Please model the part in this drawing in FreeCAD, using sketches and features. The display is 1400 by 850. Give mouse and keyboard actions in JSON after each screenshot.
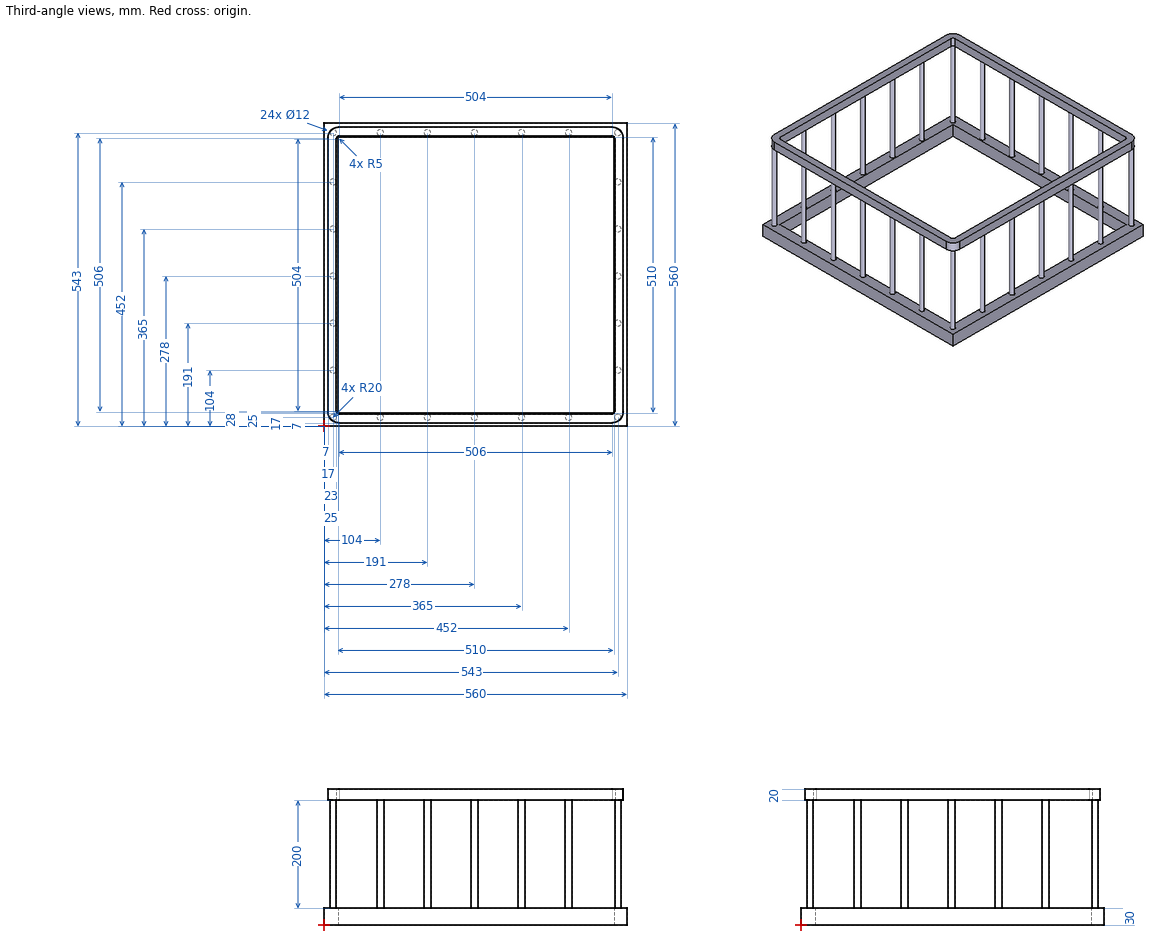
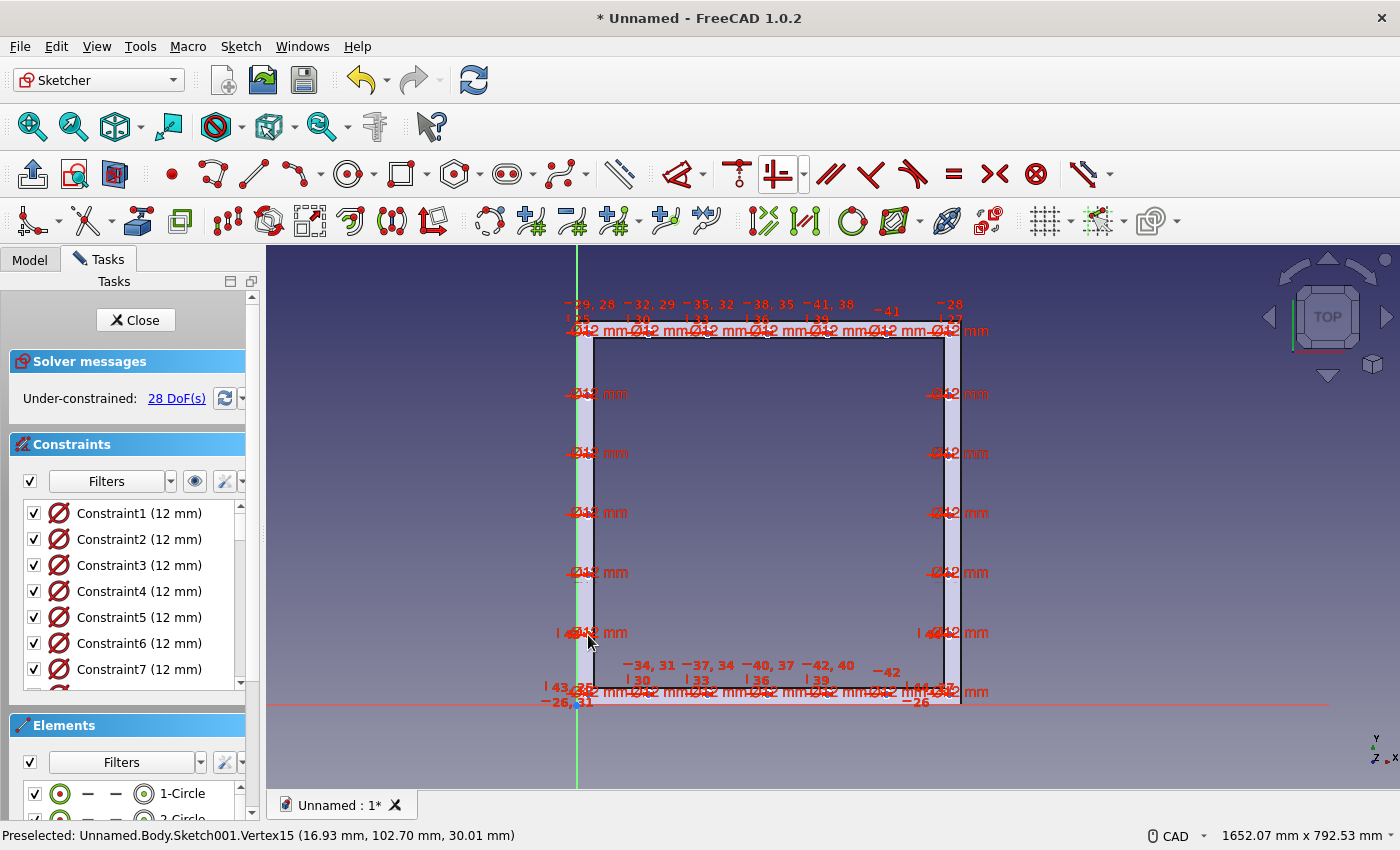
{"action": "left_click", "coordinate": [588, 575]}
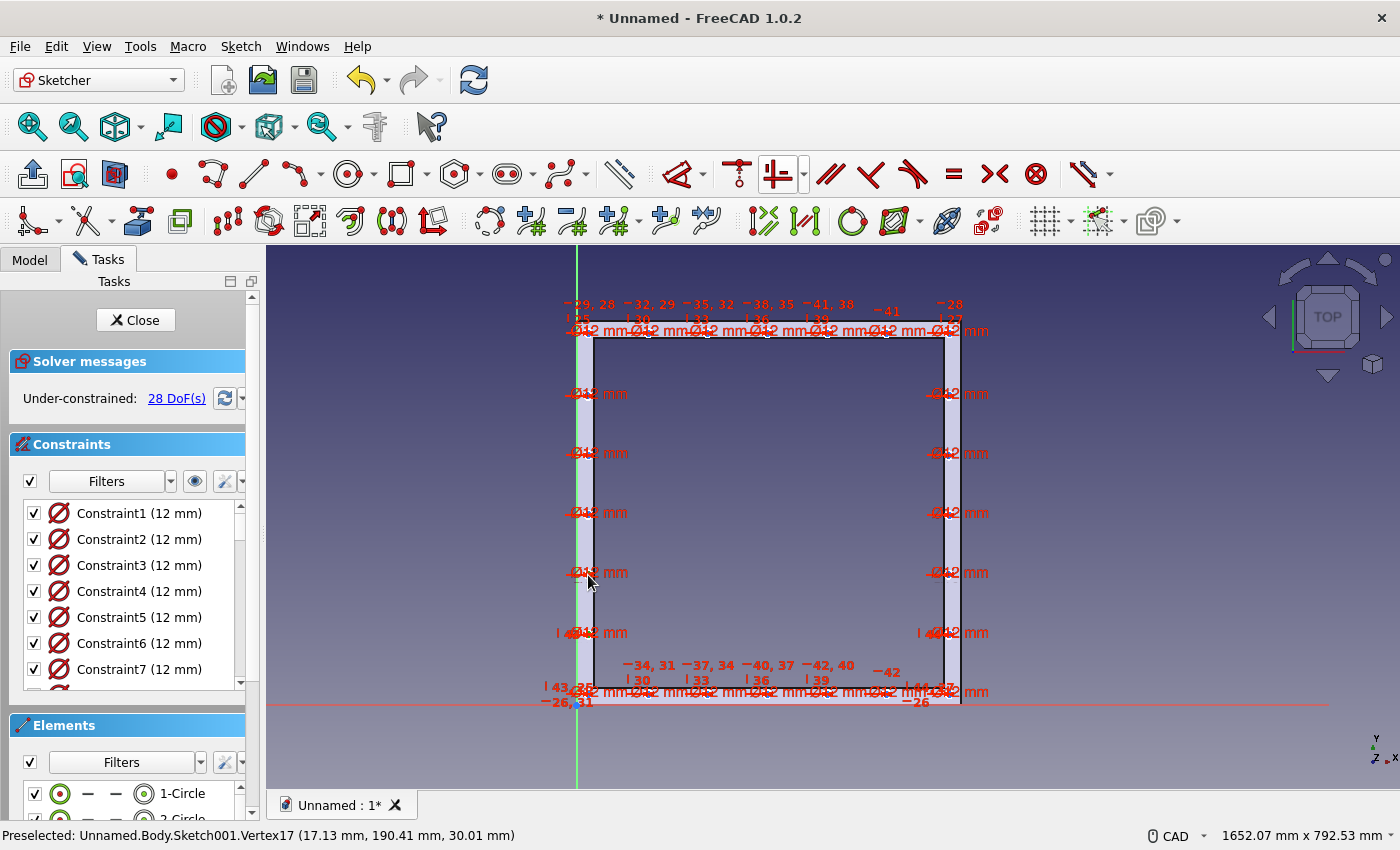
{"action": "left_click", "coordinate": [804, 174]}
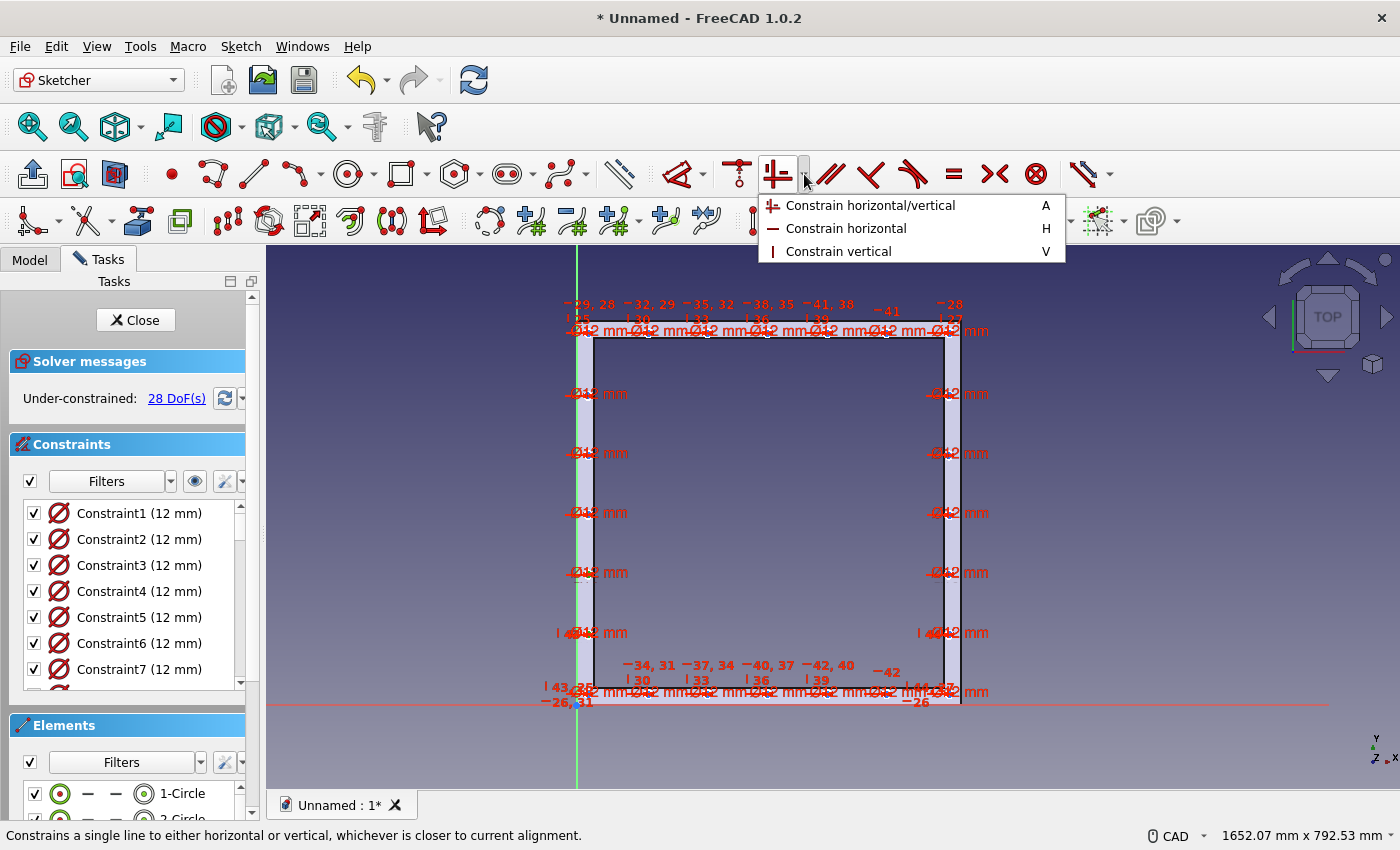
{"action": "left_click", "coordinate": [912, 252]}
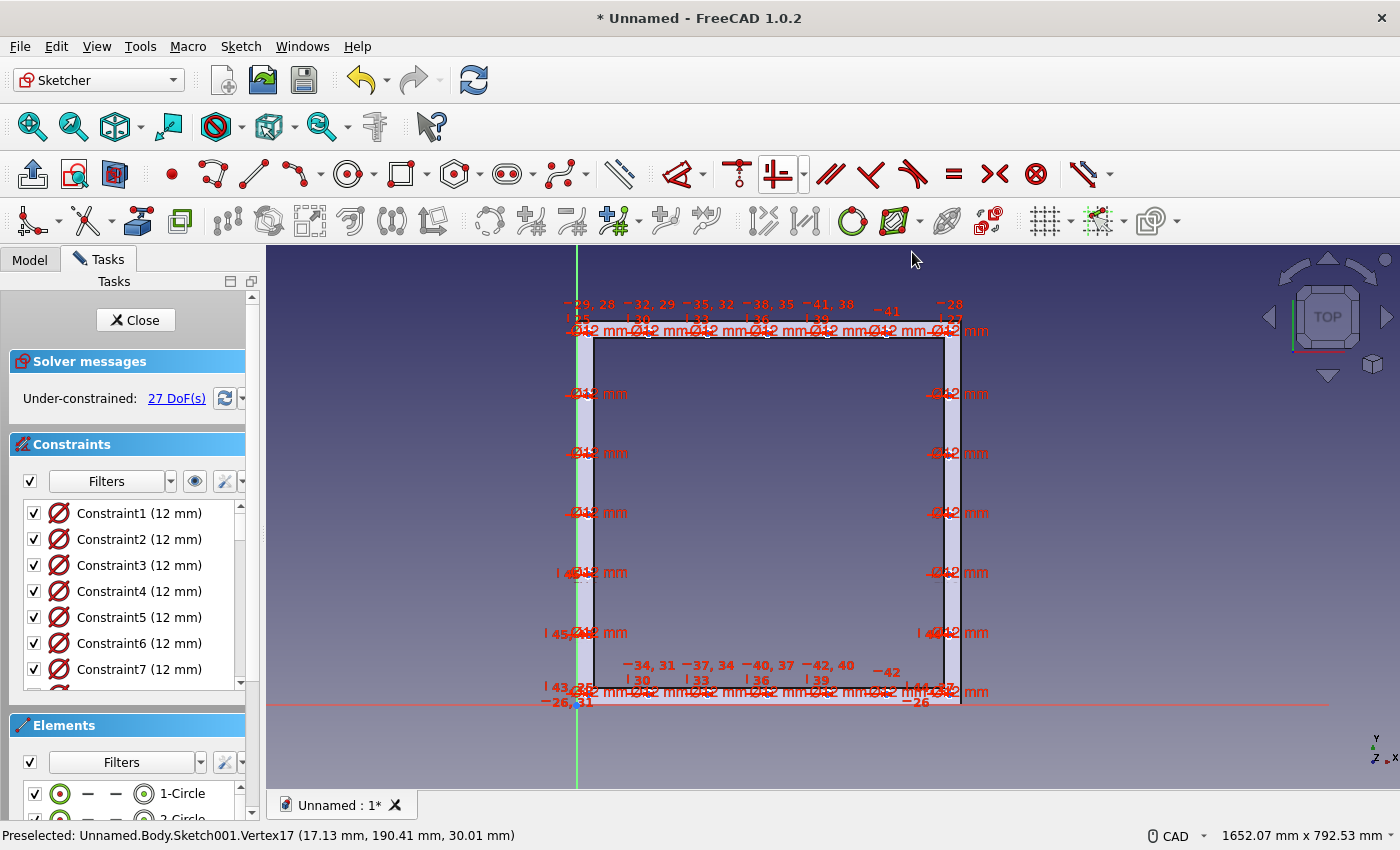
{"action": "left_click", "coordinate": [949, 635]}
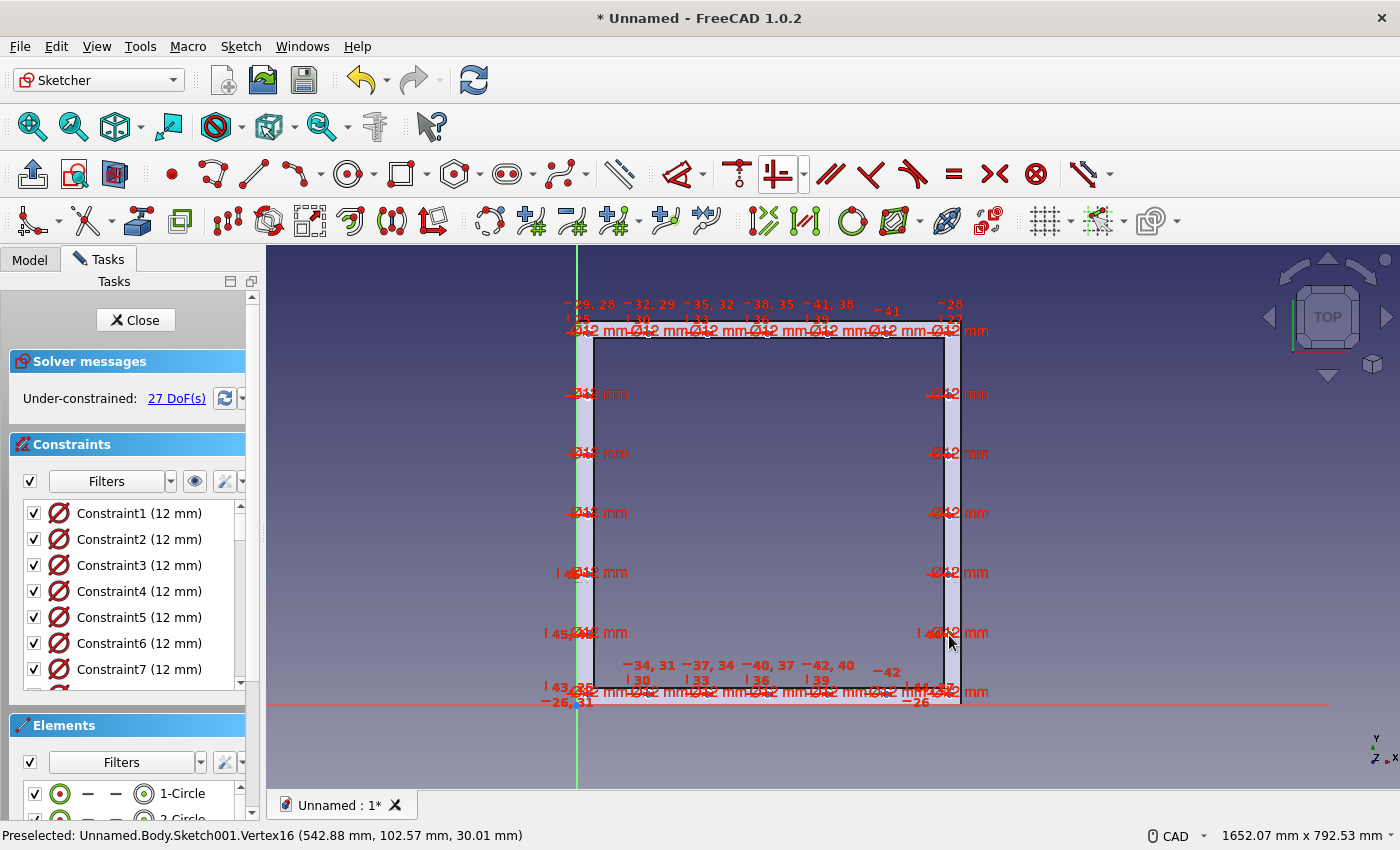
{"action": "left_click", "coordinate": [949, 575]}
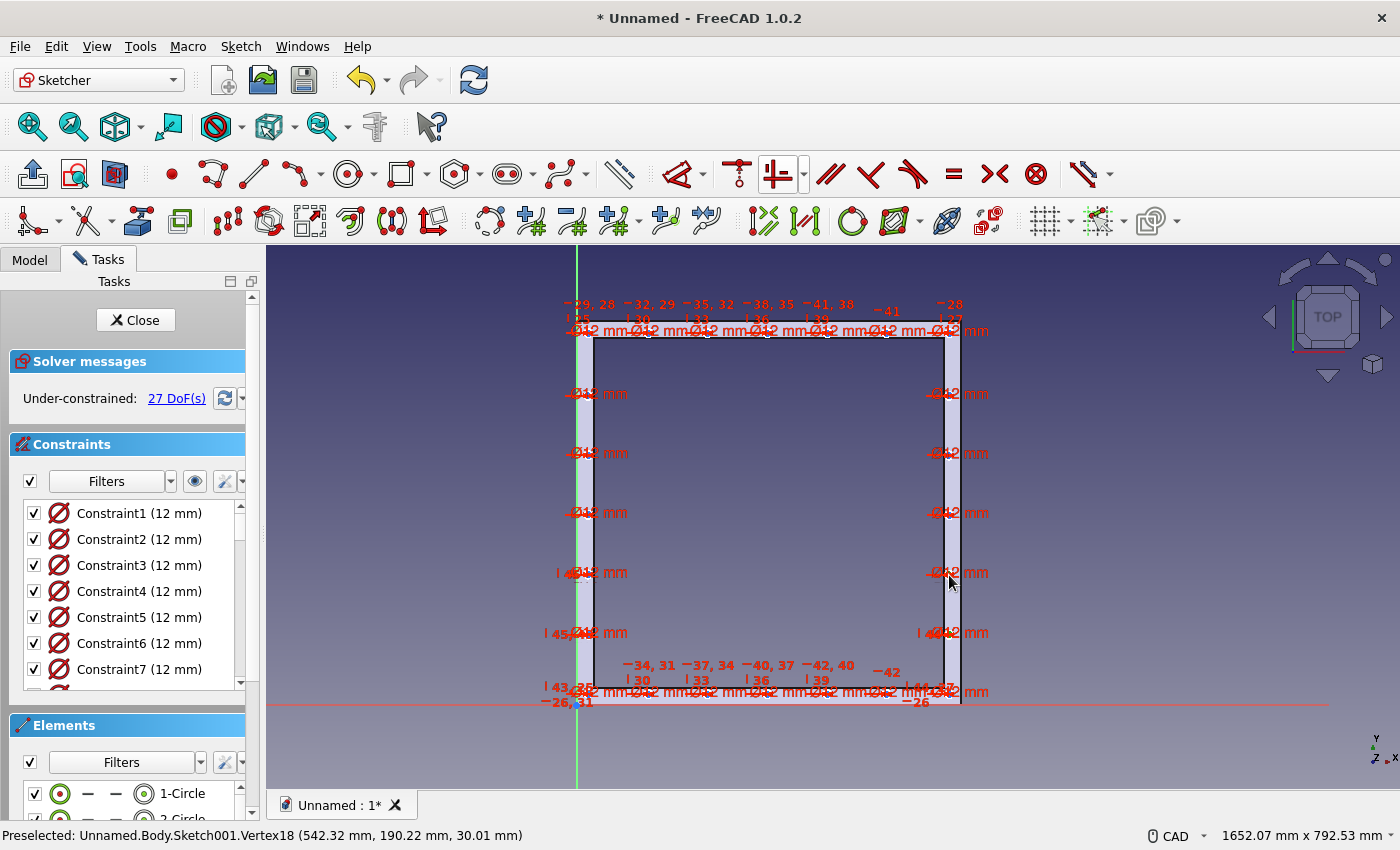
{"action": "left_click", "coordinate": [804, 174]}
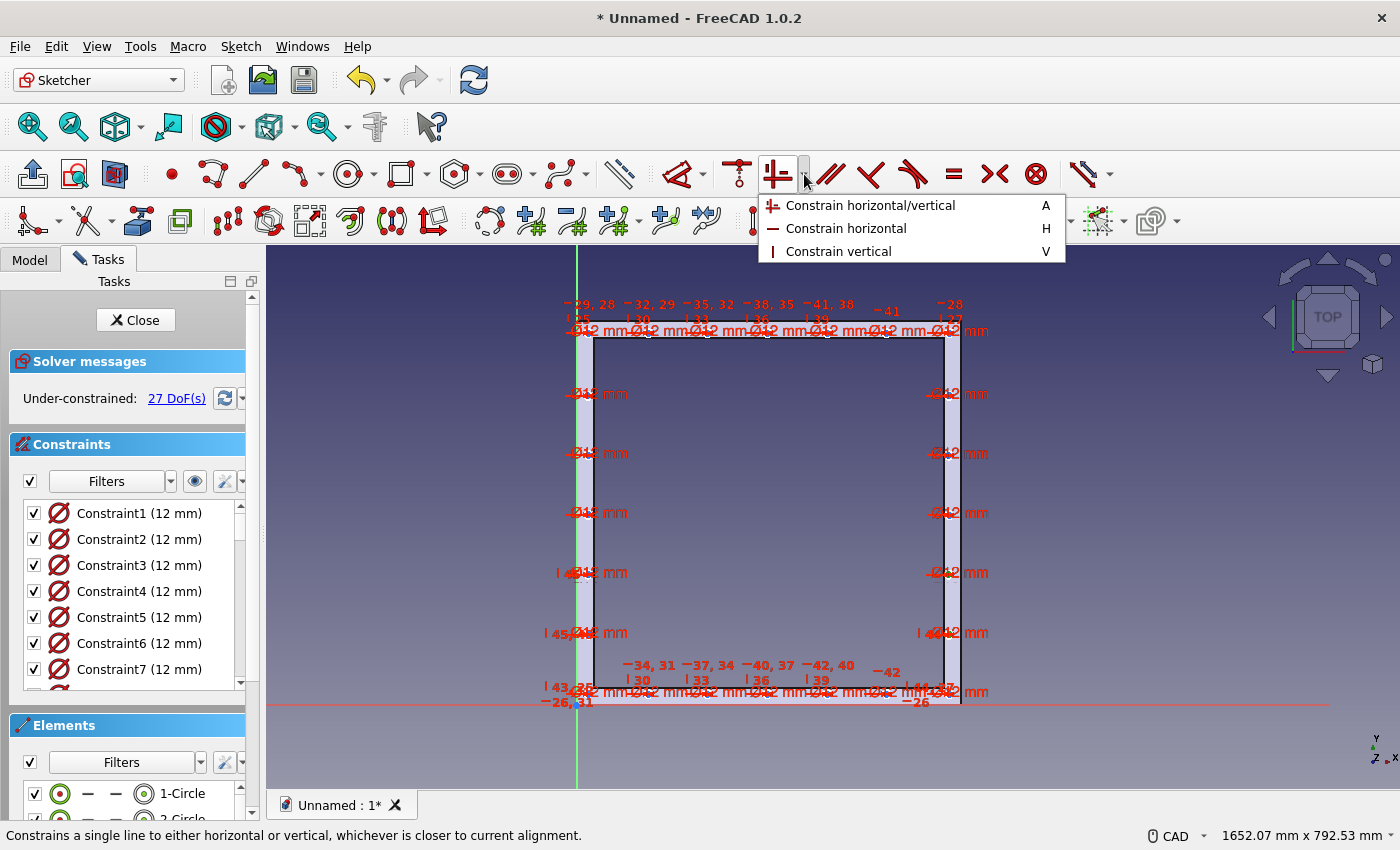
{"action": "left_click", "coordinate": [912, 252]}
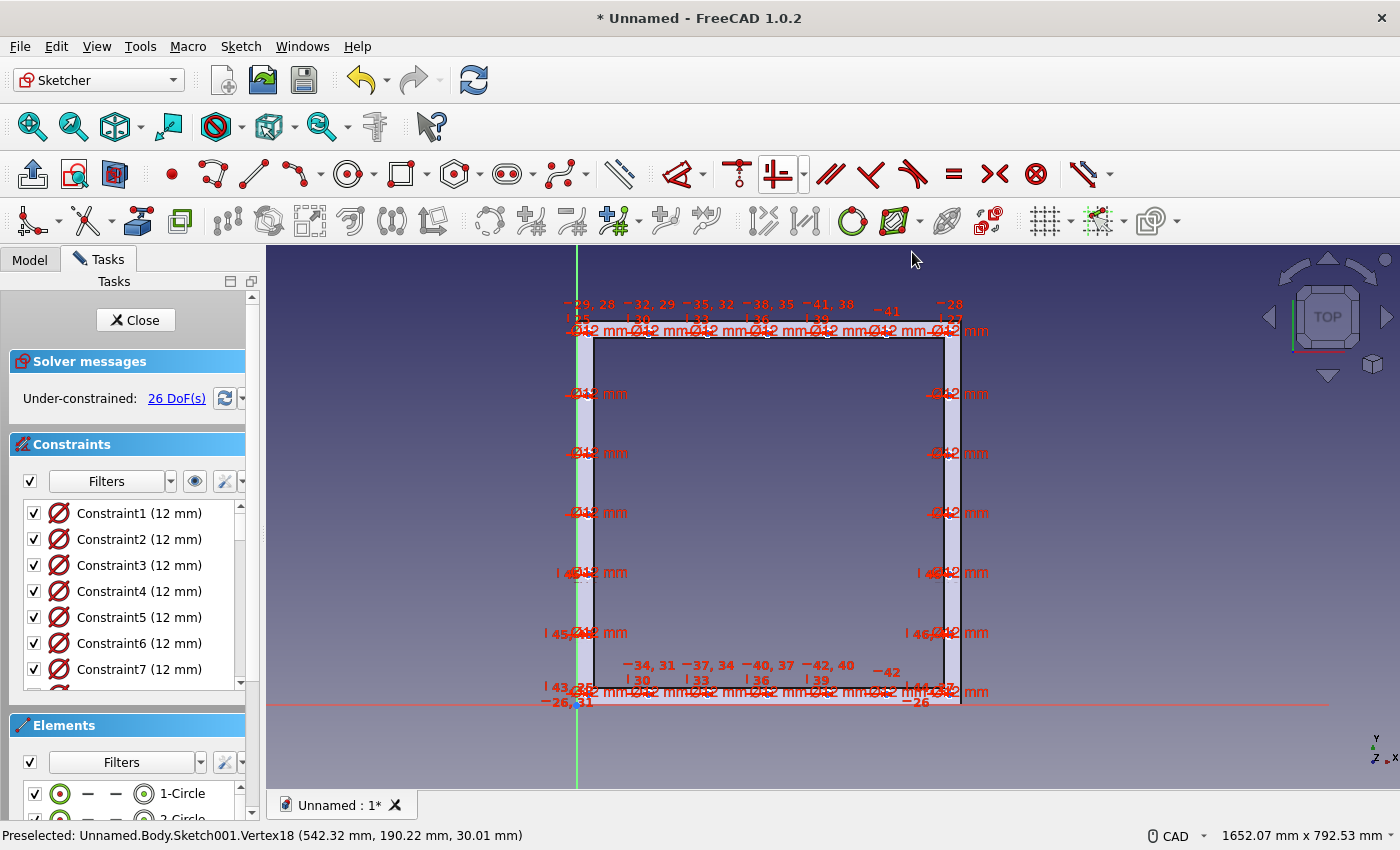
{"action": "left_click", "coordinate": [588, 575]}